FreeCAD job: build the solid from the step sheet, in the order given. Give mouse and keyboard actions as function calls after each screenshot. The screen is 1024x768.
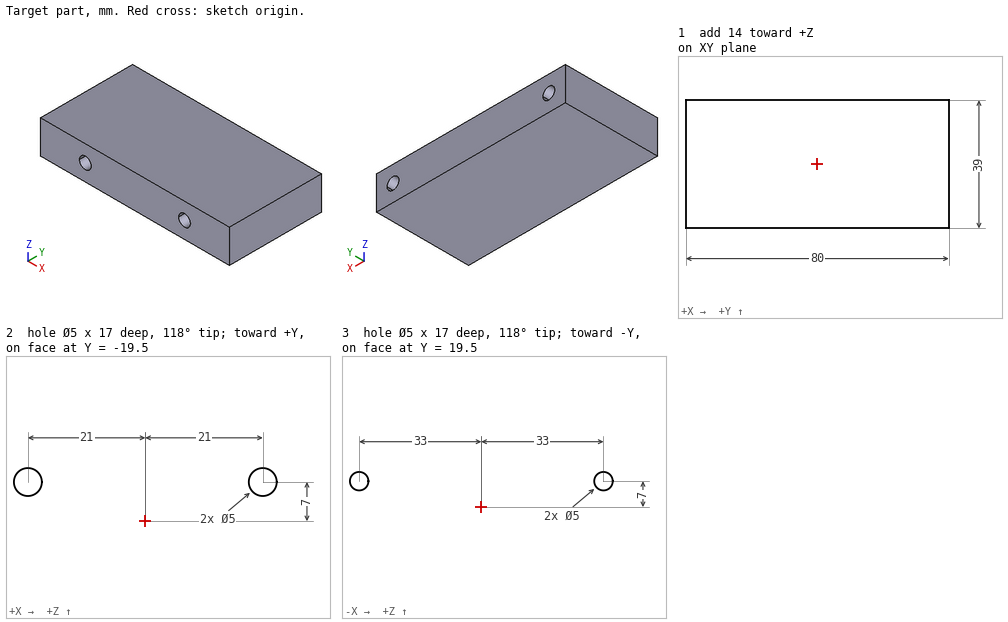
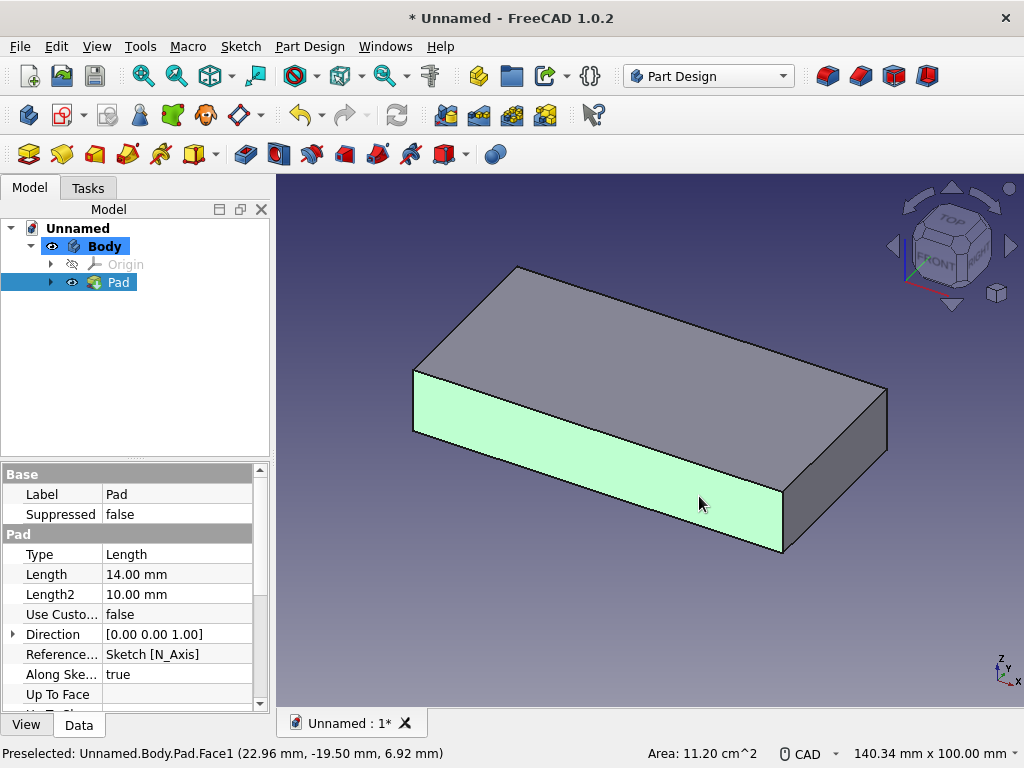
click(62, 116)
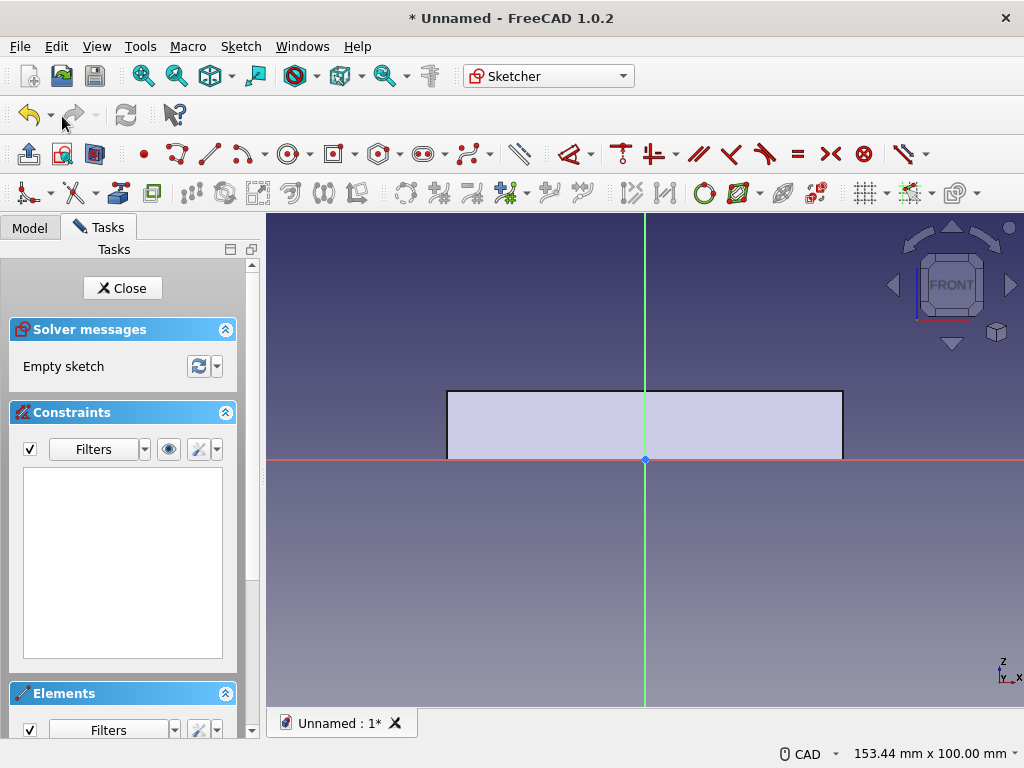
scroll(728, 408, up, 3)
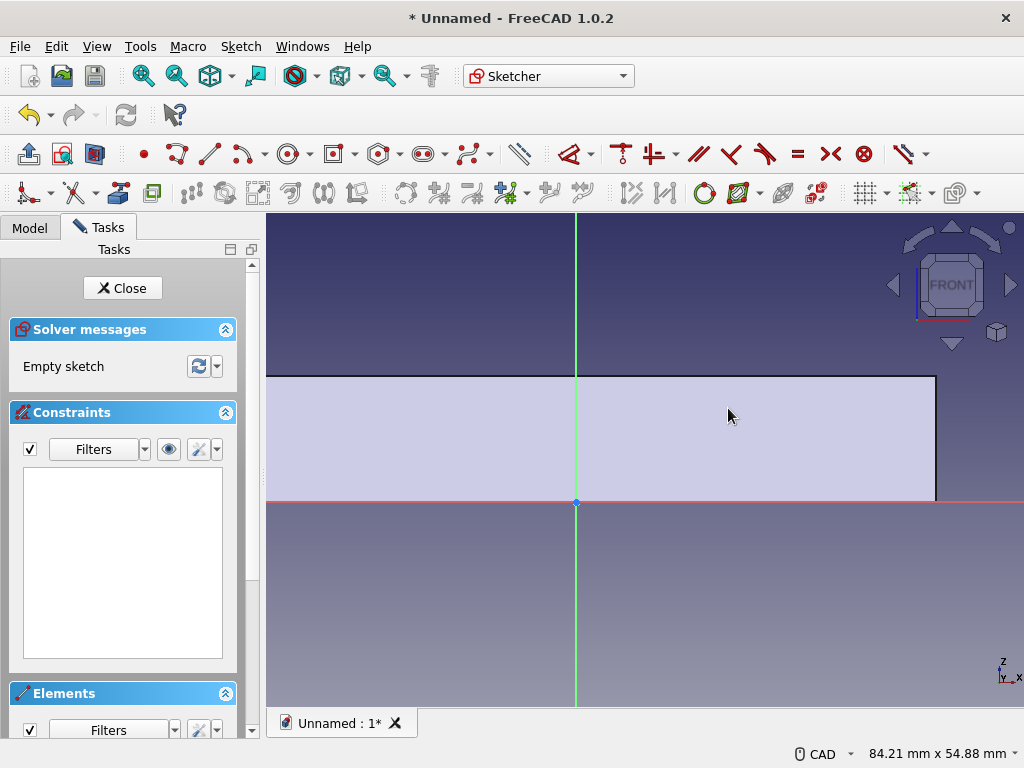
click(288, 154)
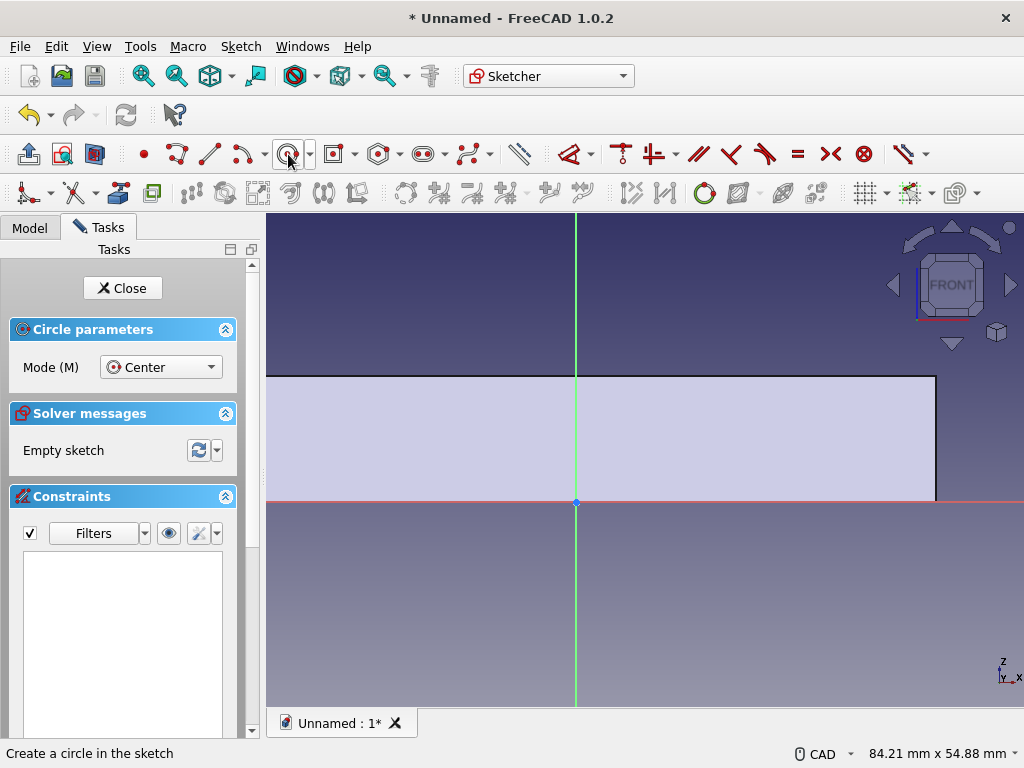
click(765, 439)
move(781, 424)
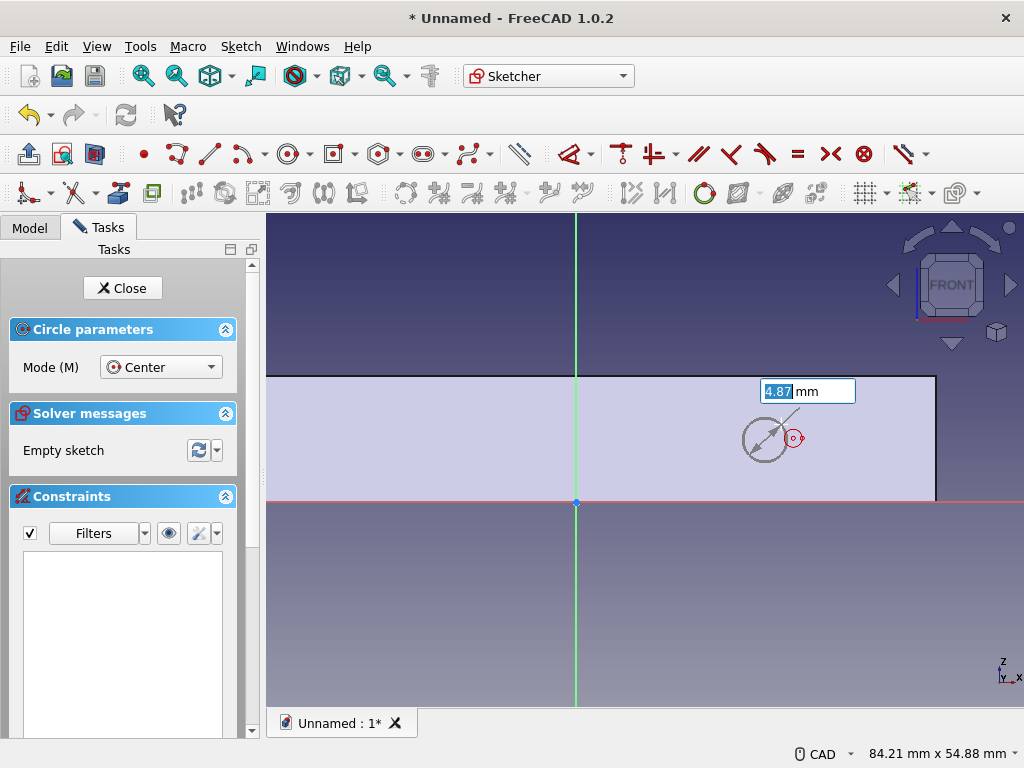
text(5)
key(Return)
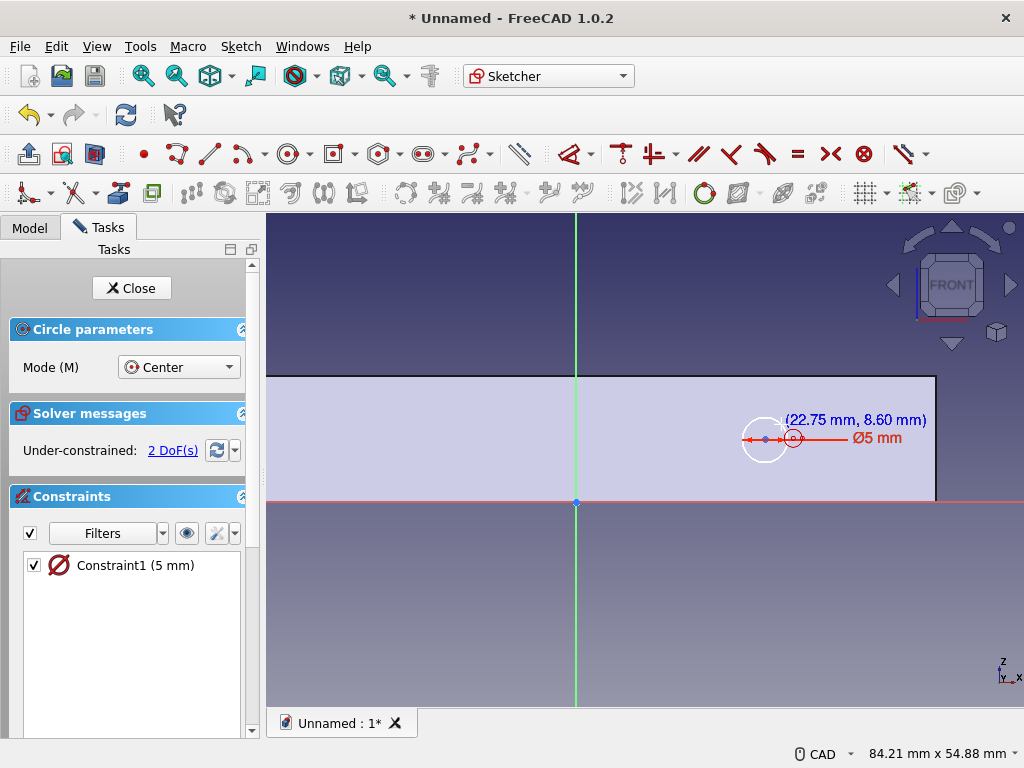
click(387, 439)
move(403, 424)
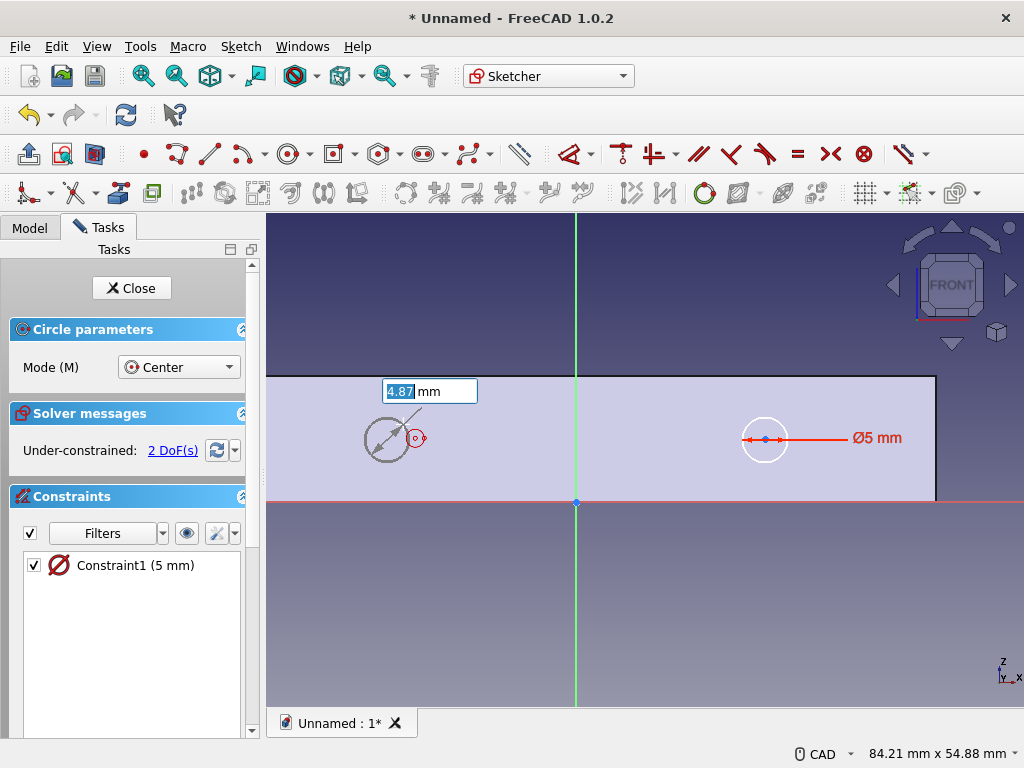
text(5)
key(Return)
key(Escape)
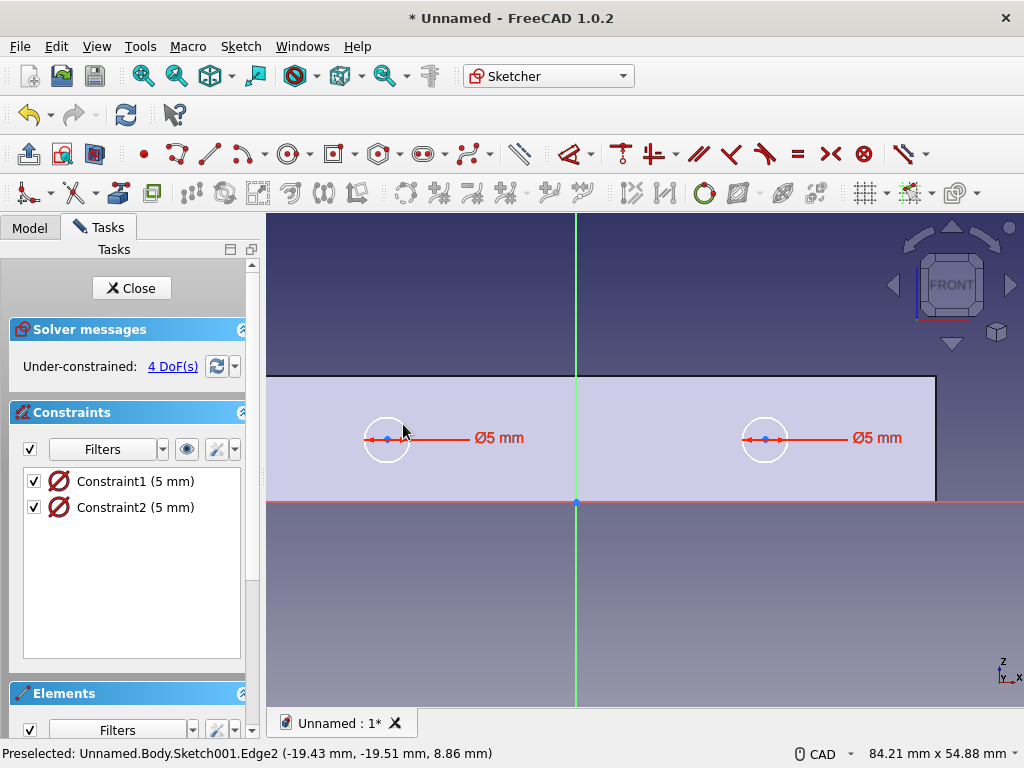
click(765, 440)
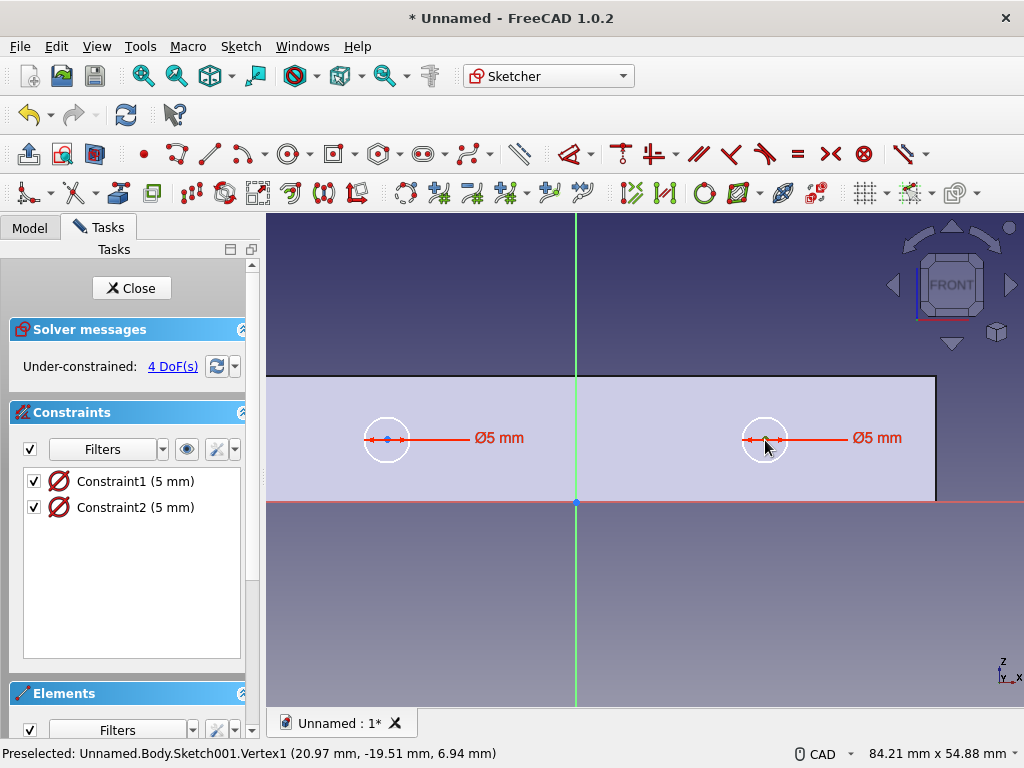
click(387, 440)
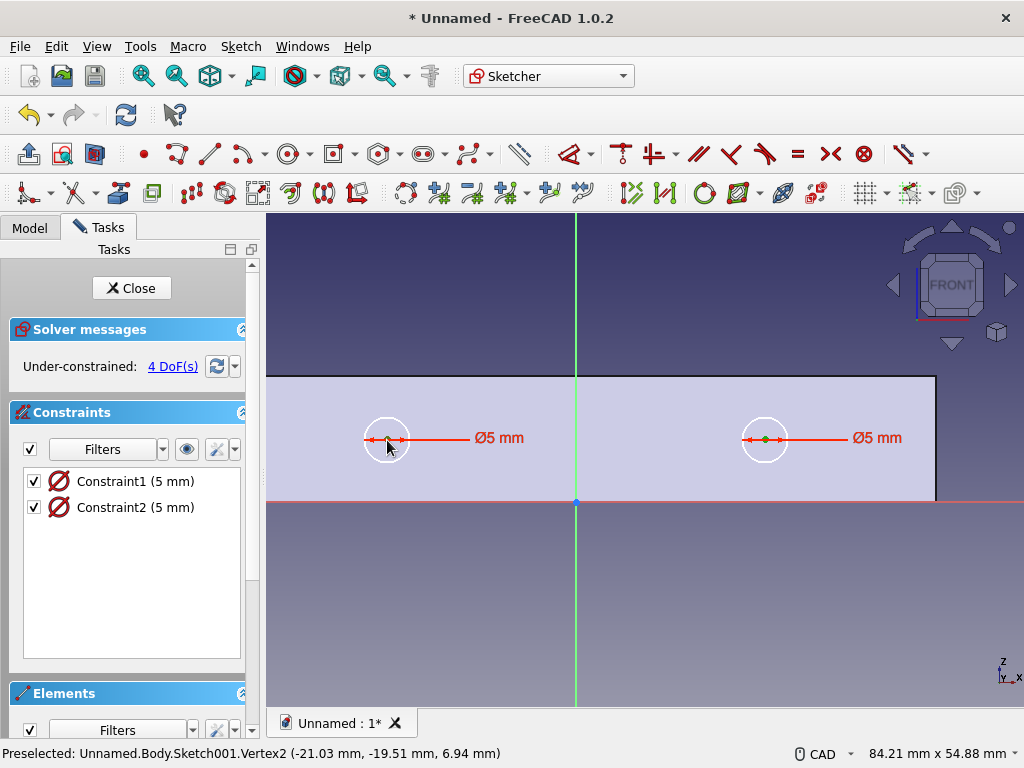
click(676, 154)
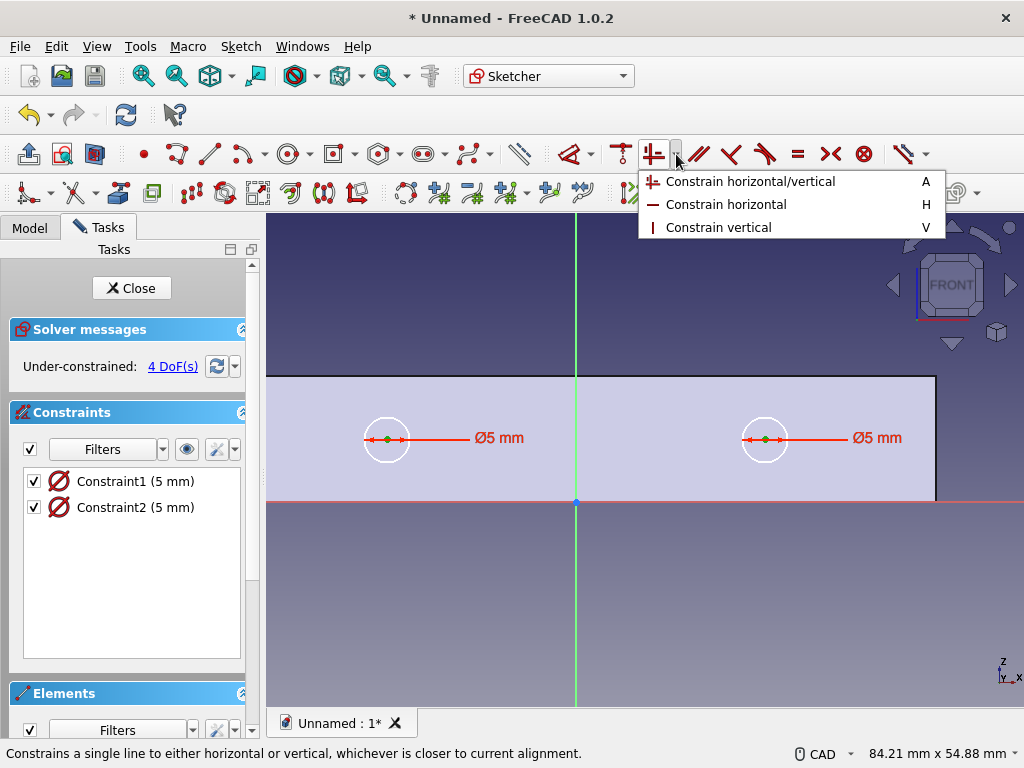
click(792, 204)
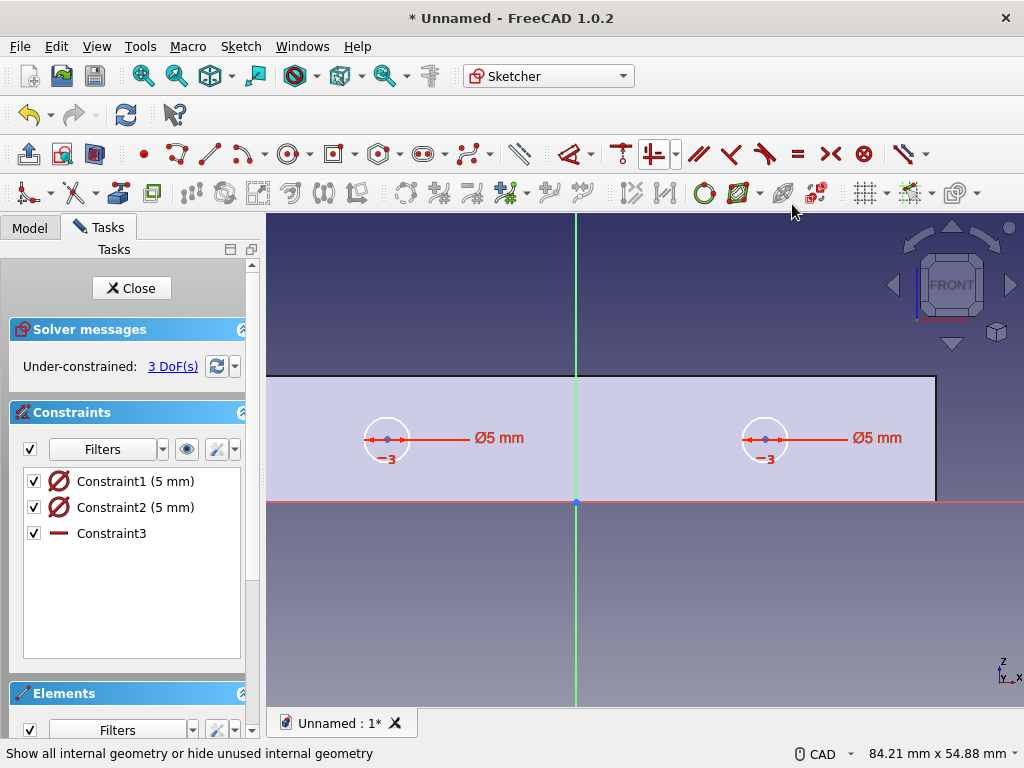
click(568, 154)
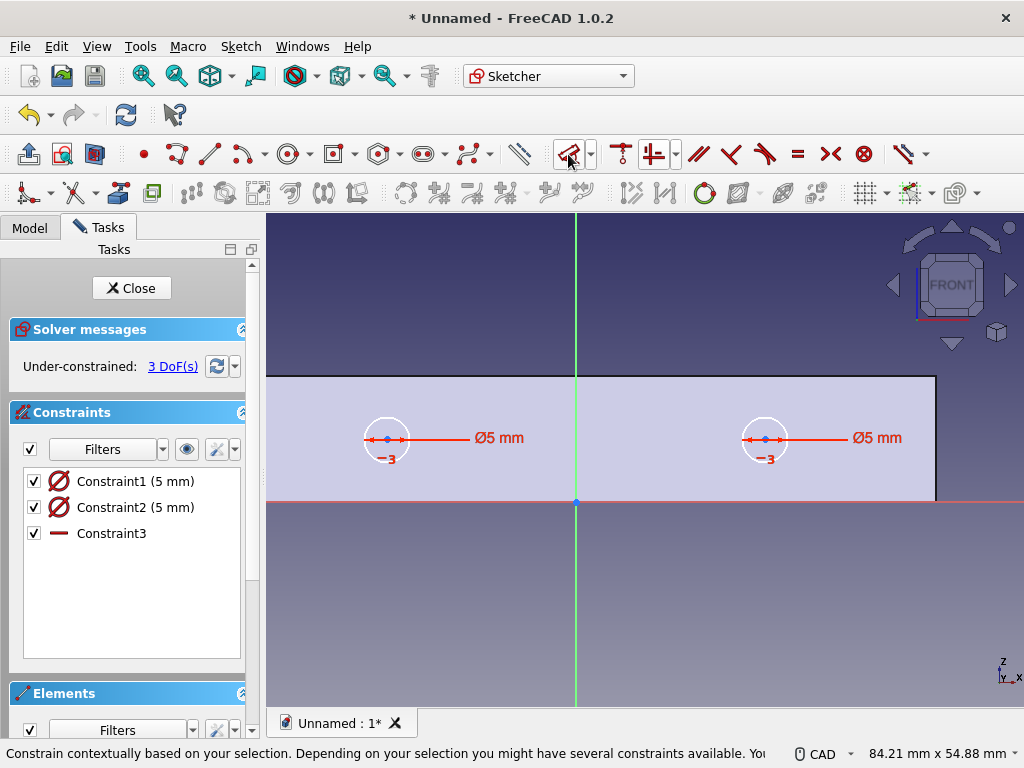
click(765, 440)
click(799, 471)